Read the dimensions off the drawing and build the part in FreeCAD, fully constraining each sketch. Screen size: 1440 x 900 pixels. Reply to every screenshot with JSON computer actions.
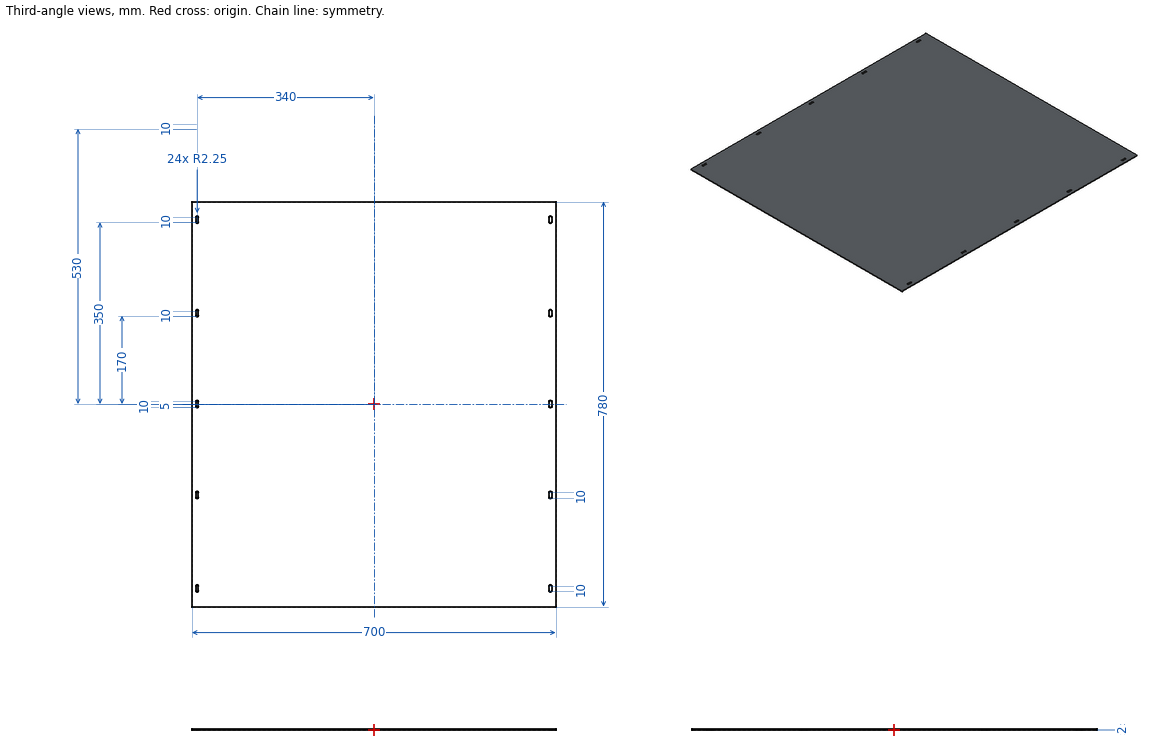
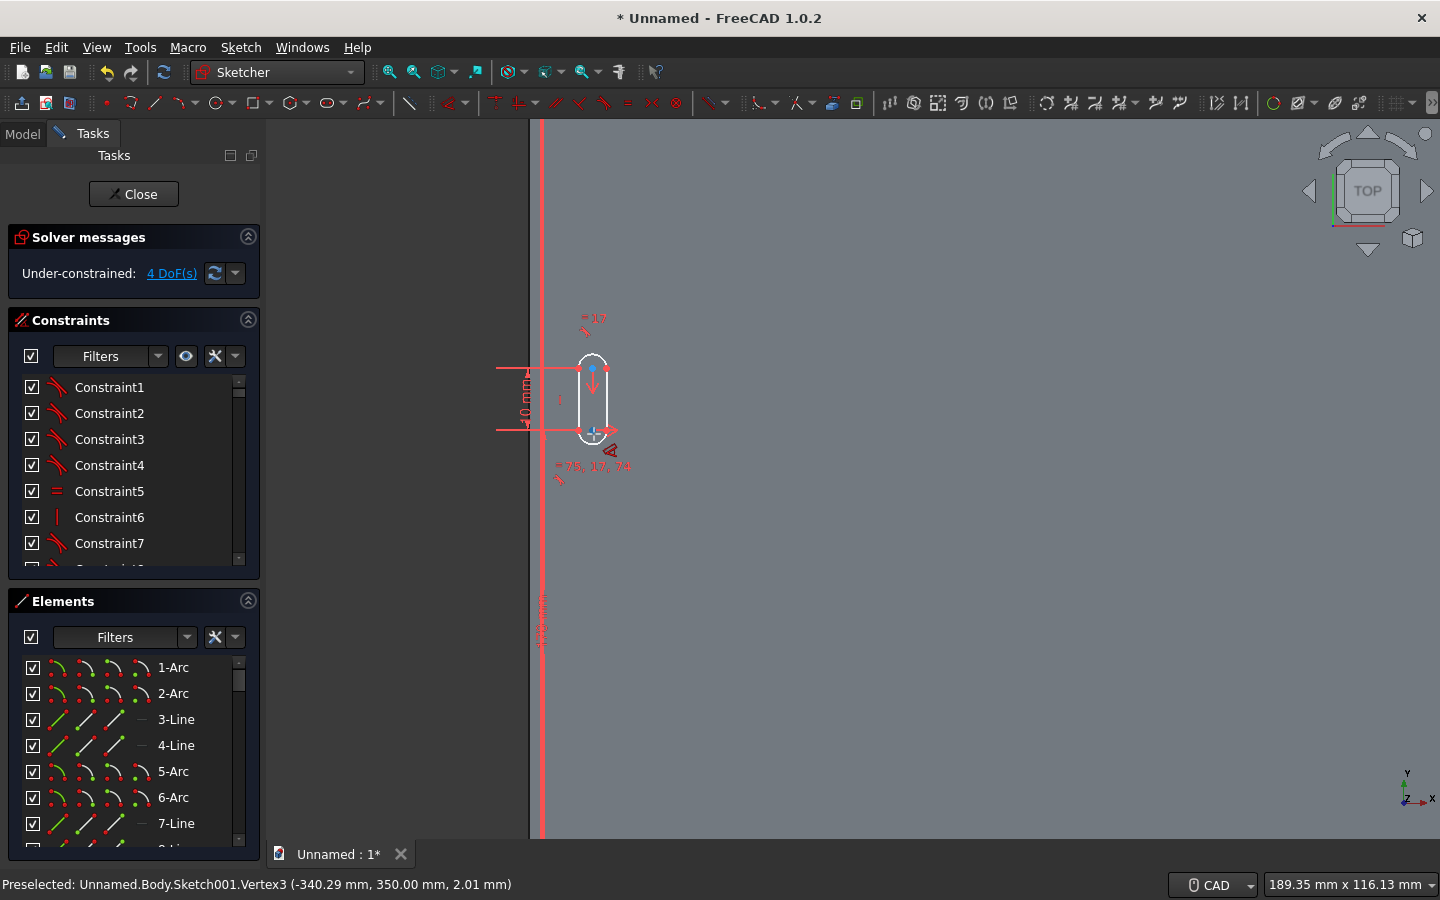
{"action": "left_click", "coordinate": [593, 430]}
{"action": "left_click", "coordinate": [934, 396]}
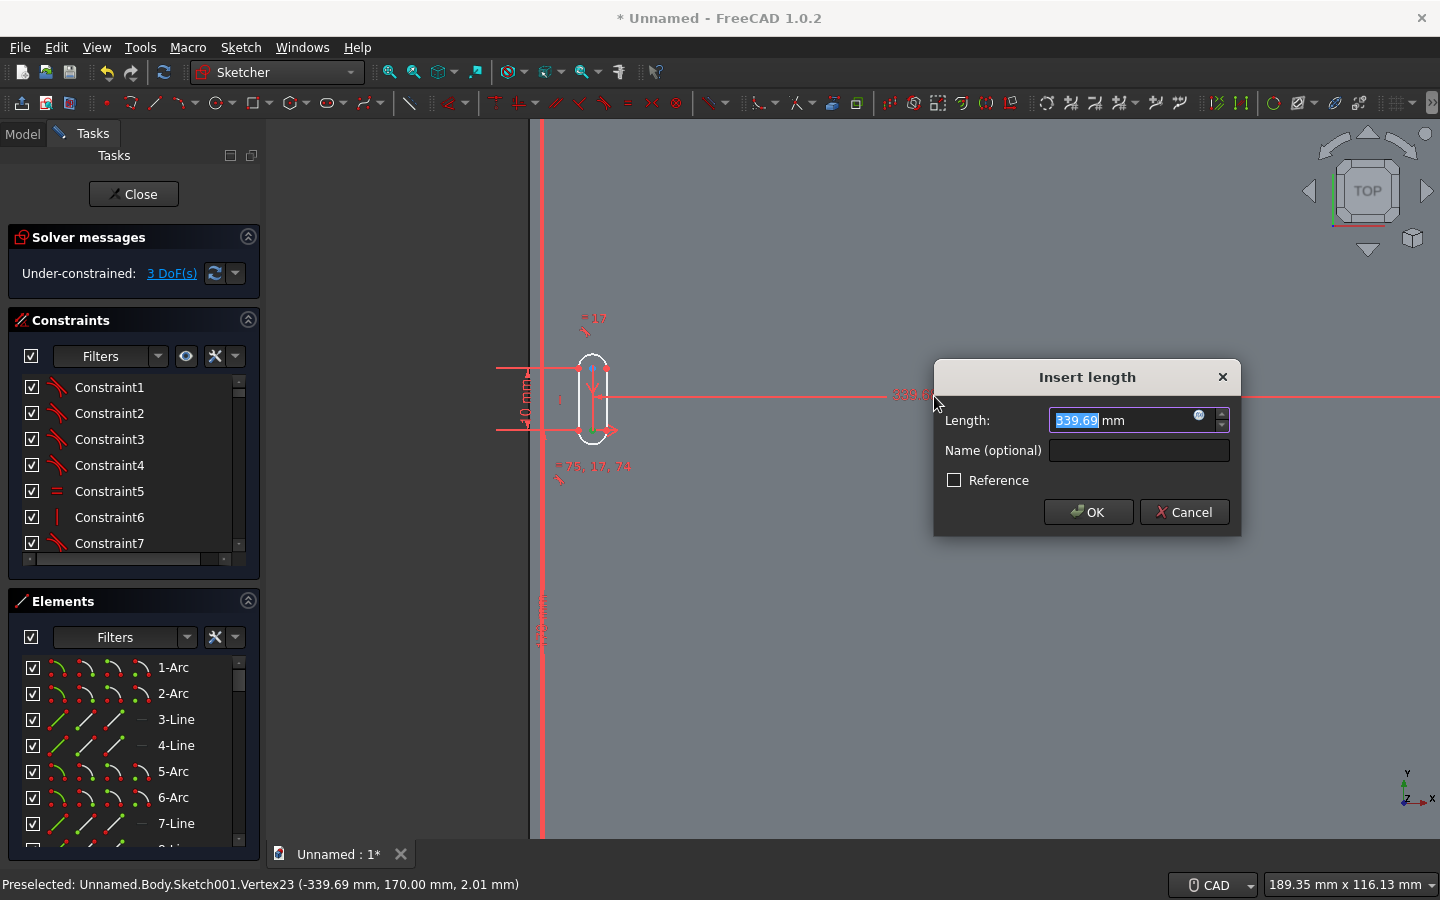
{"action": "type", "text": "340"}
{"action": "key", "text": "Return"}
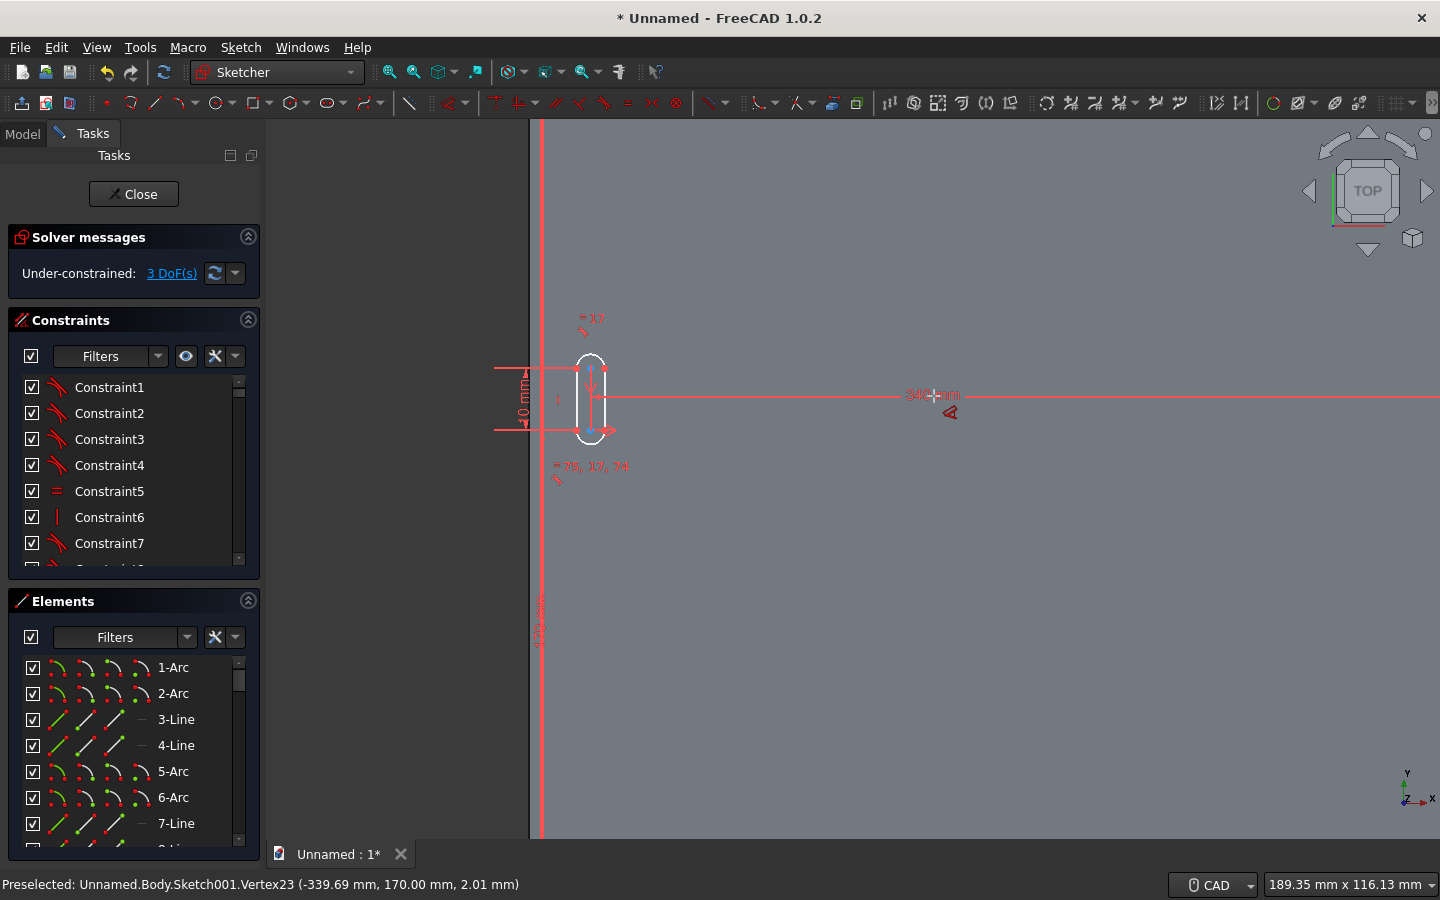
{"action": "scroll", "coordinate": [594, 434], "scroll_direction": "down", "scroll_amount": 12}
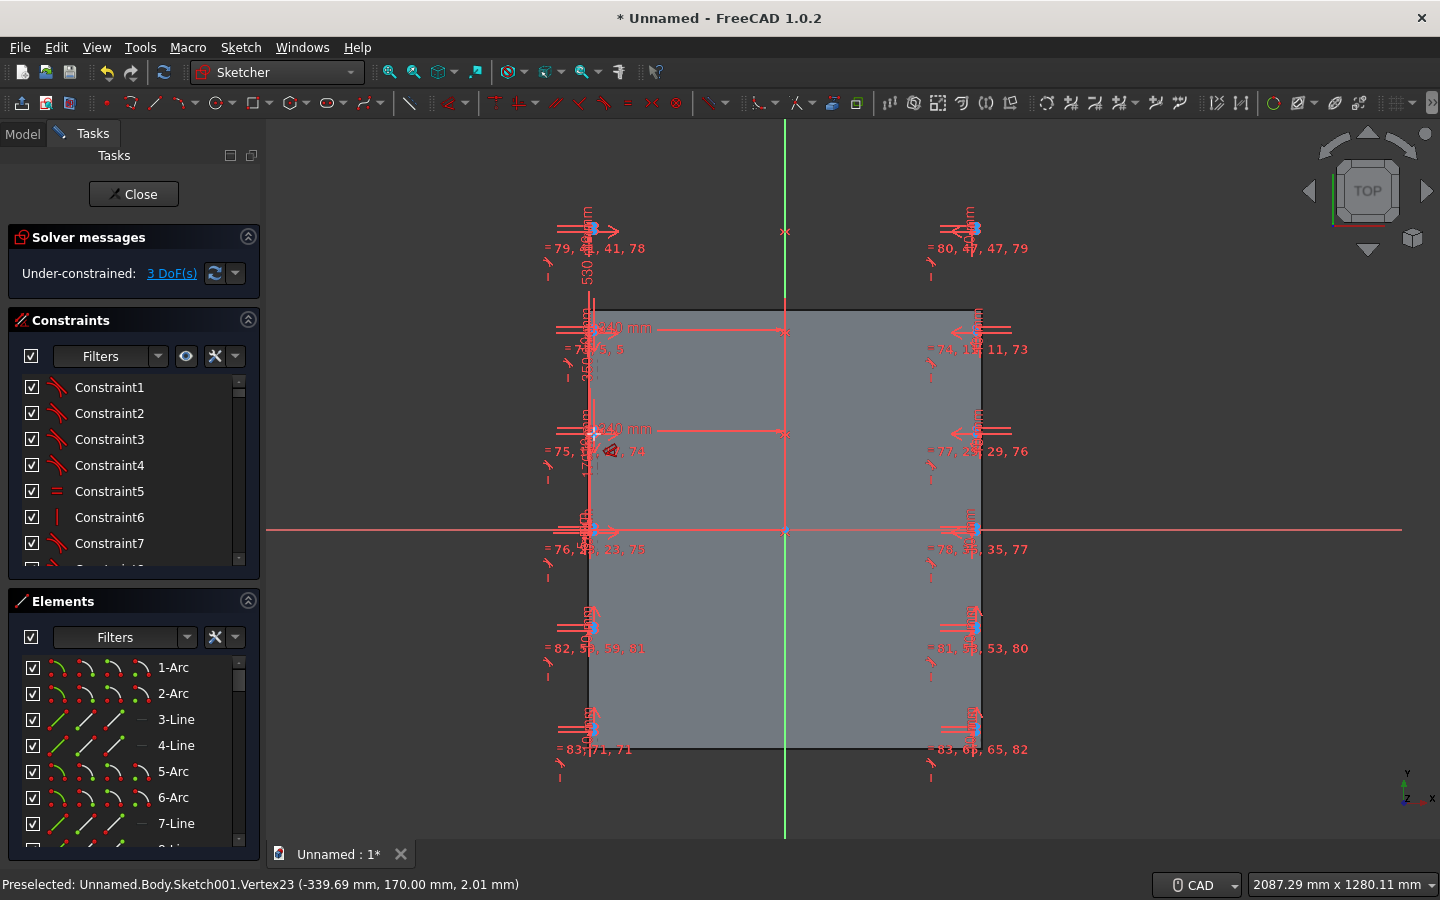
{"action": "scroll", "coordinate": [594, 533], "scroll_direction": "up", "scroll_amount": 12}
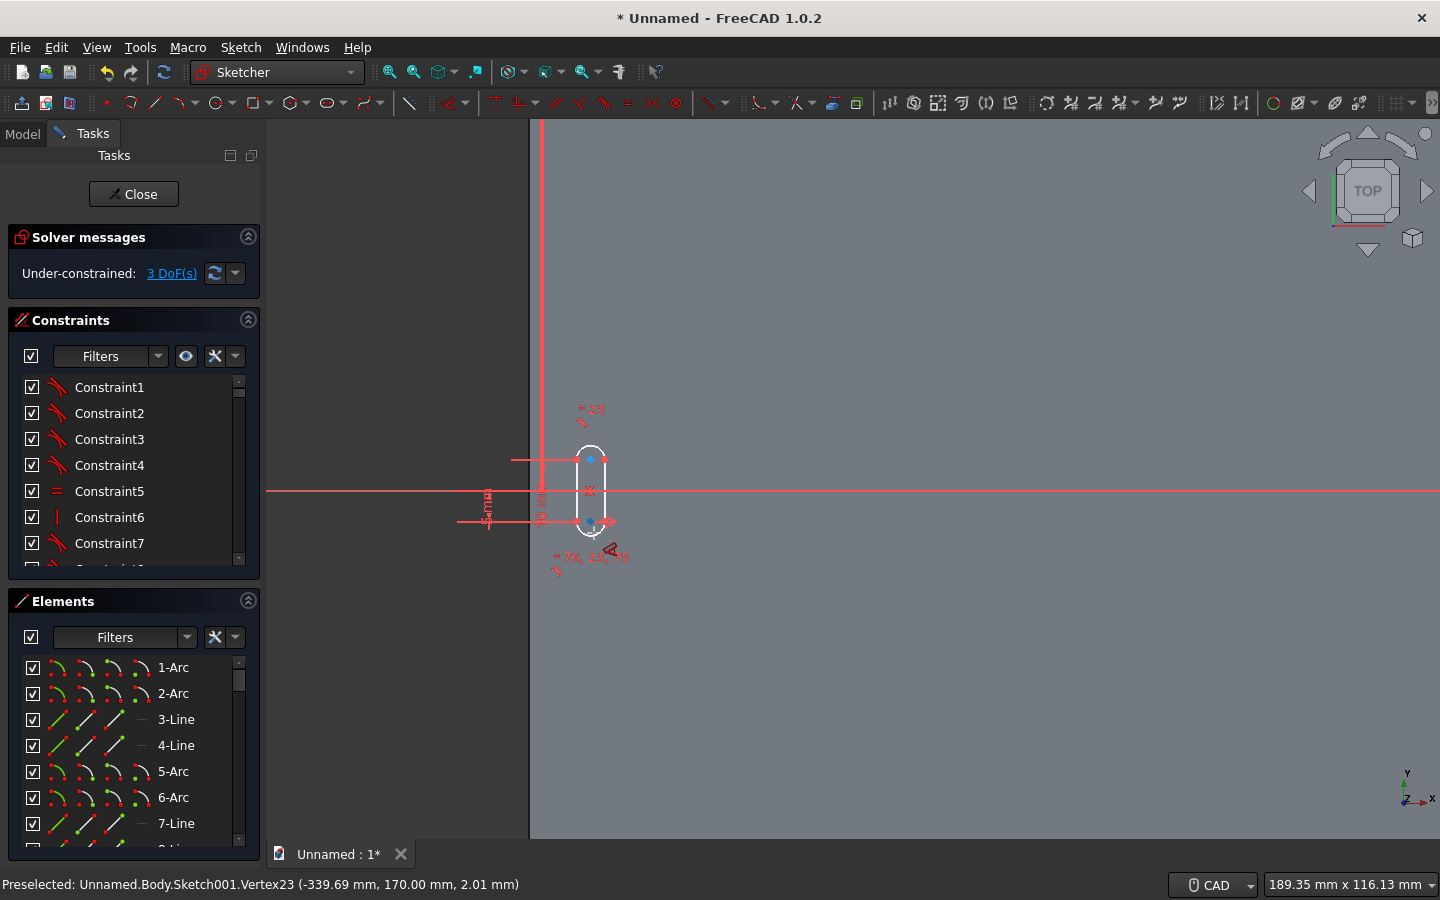
{"action": "left_click", "coordinate": [591, 522]}
{"action": "left_click", "coordinate": [933, 556]}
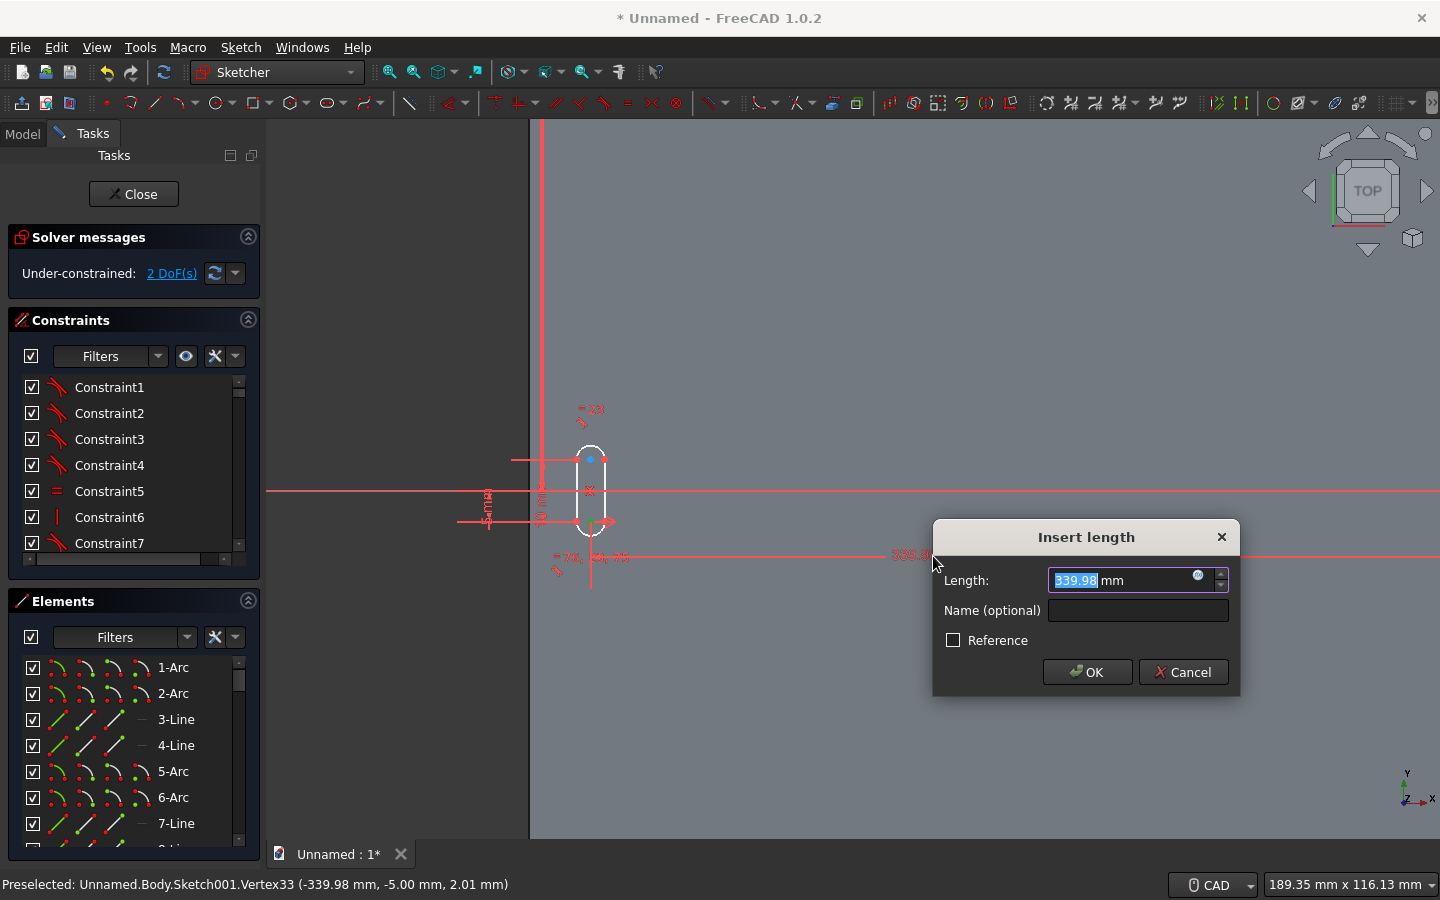
{"action": "type", "text": "340"}
{"action": "key", "text": "Return"}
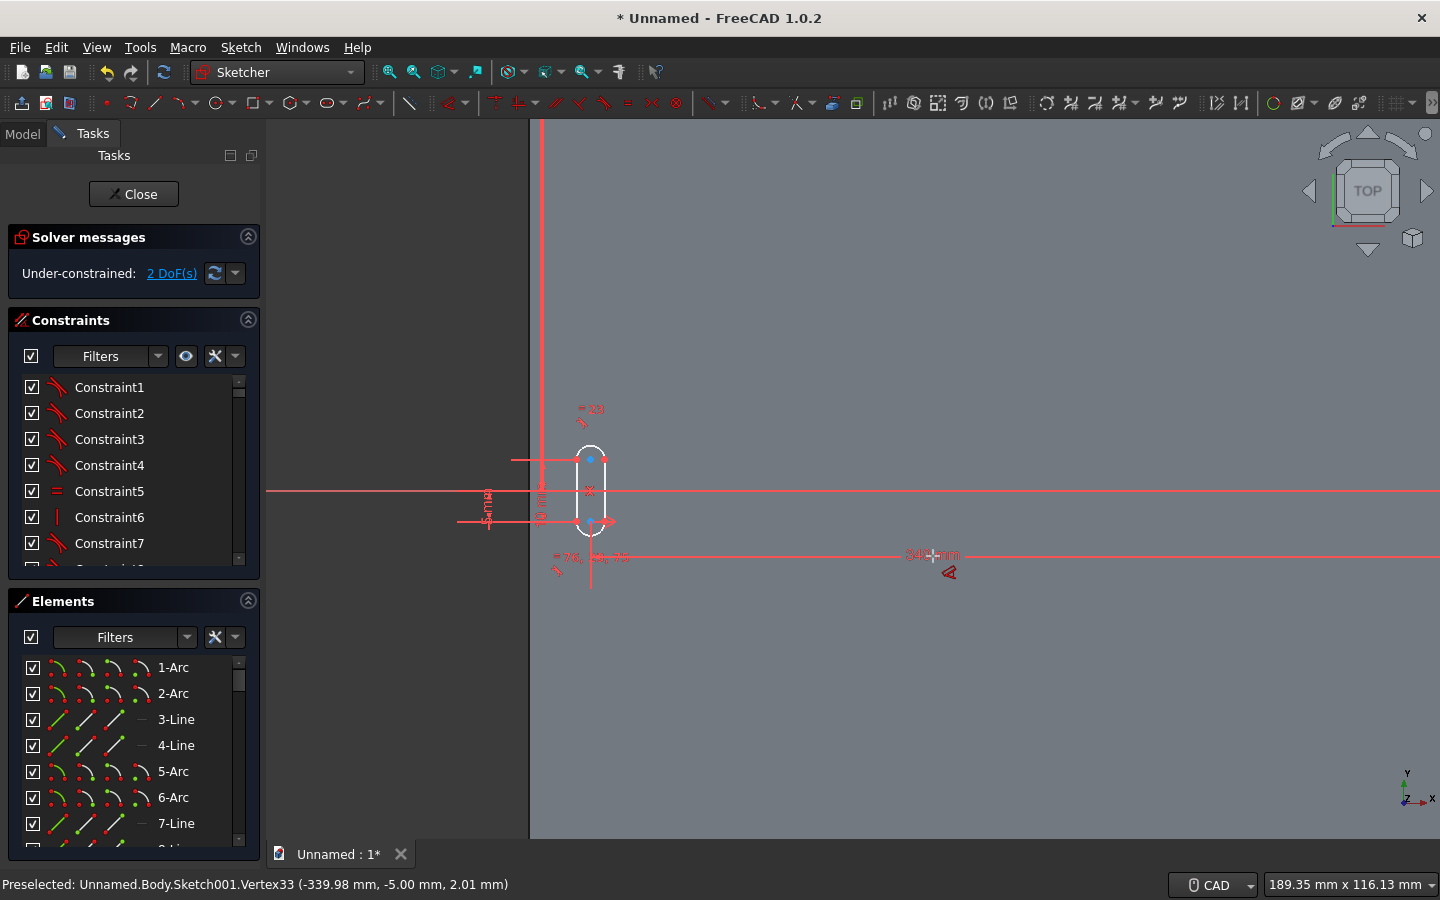
{"action": "scroll", "coordinate": [594, 533], "scroll_direction": "down", "scroll_amount": 12}